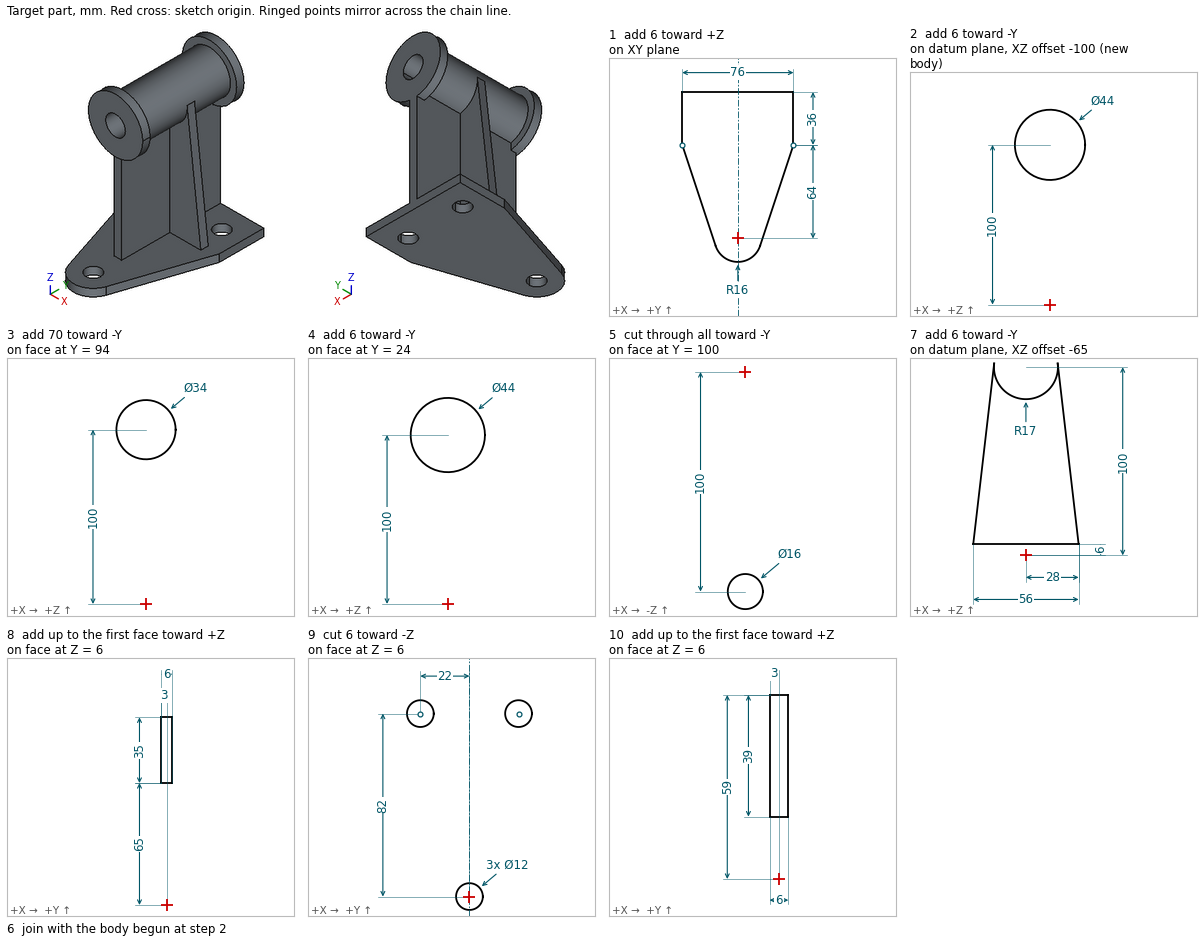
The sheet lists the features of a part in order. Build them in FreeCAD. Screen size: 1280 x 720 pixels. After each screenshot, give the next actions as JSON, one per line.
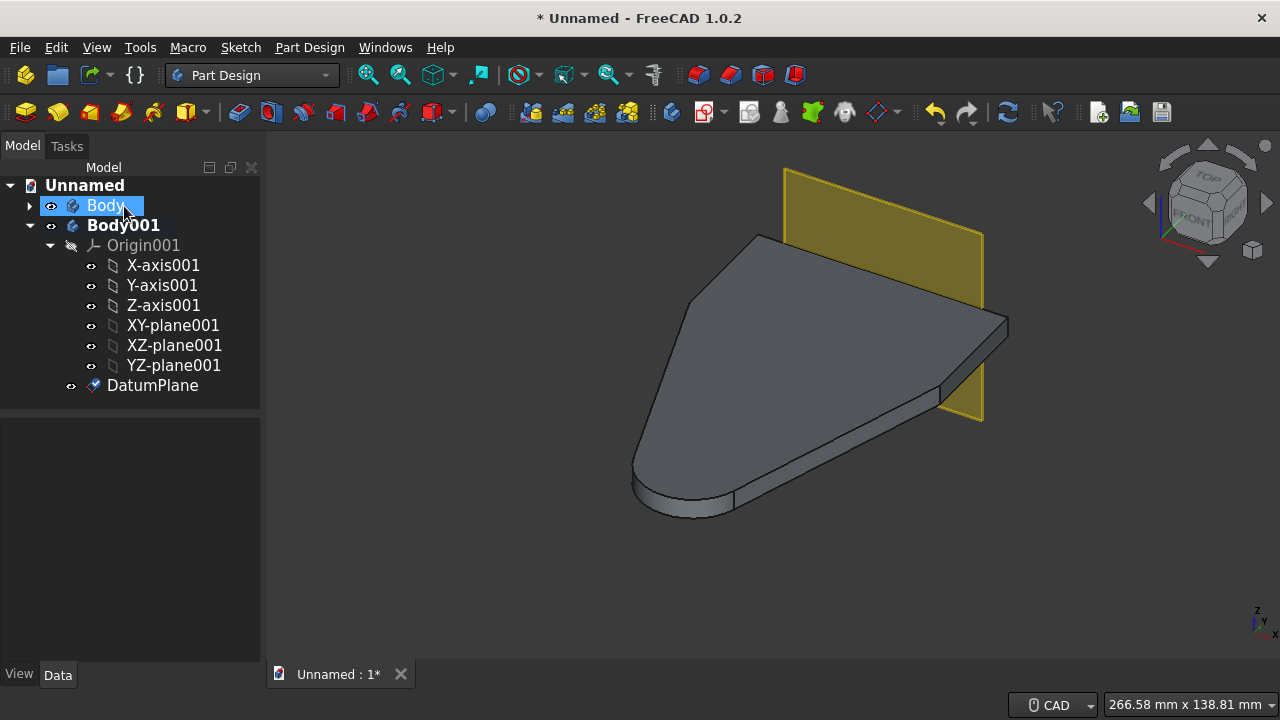
{"action": "left_click", "coordinate": [116, 386]}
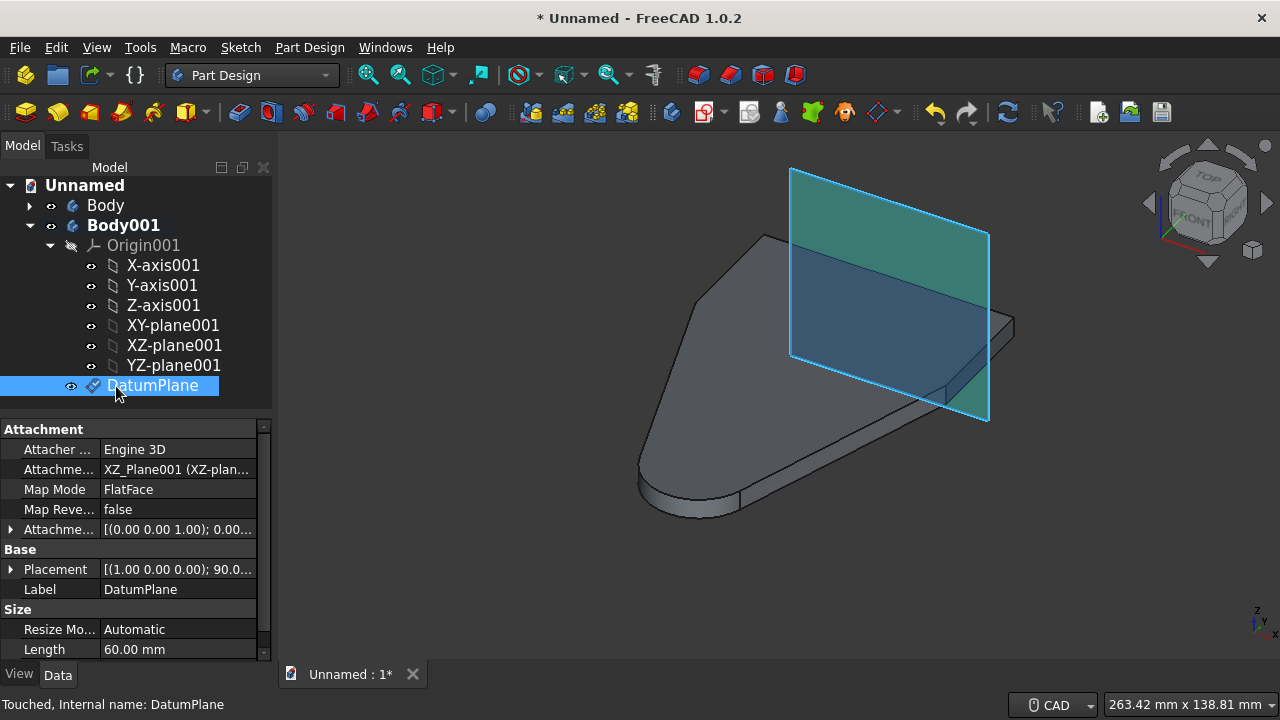
{"action": "left_click", "coordinate": [704, 112]}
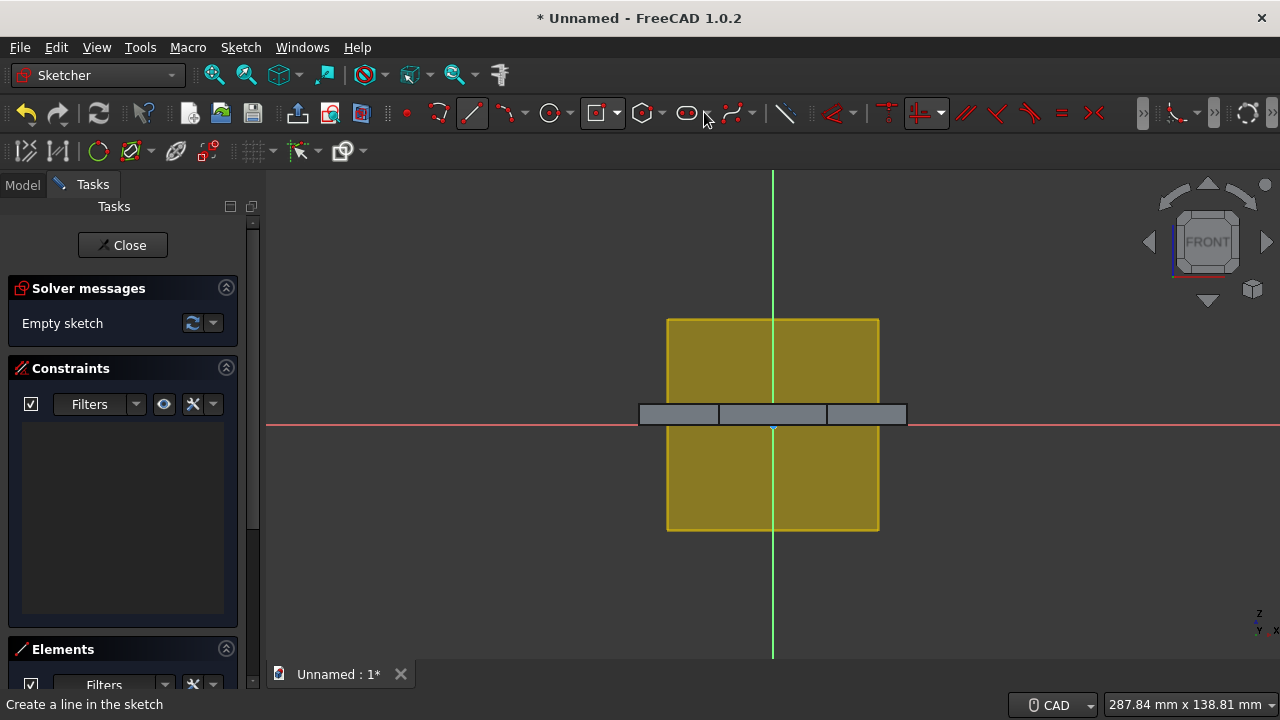
{"action": "scroll", "coordinate": [704, 414], "scroll_direction": "down", "scroll_amount": 5}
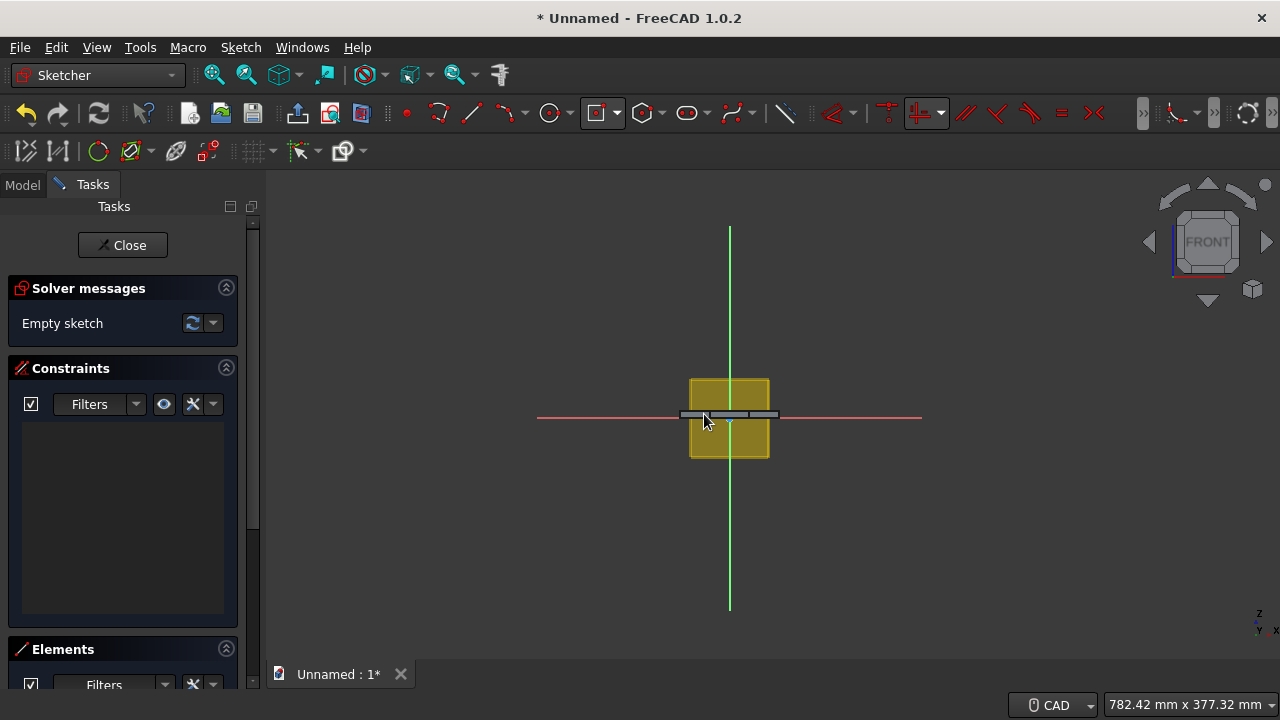
{"action": "scroll", "coordinate": [736, 257], "scroll_direction": "up", "scroll_amount": 8}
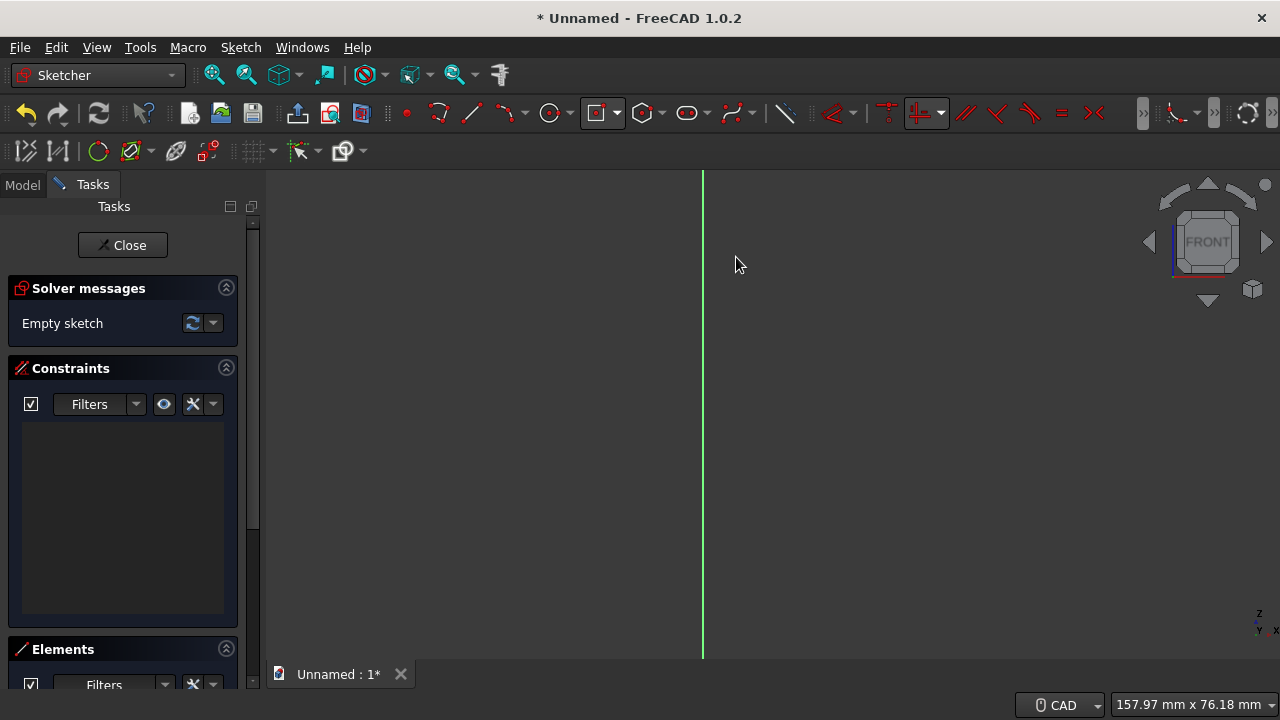
{"action": "key", "text": "g c"}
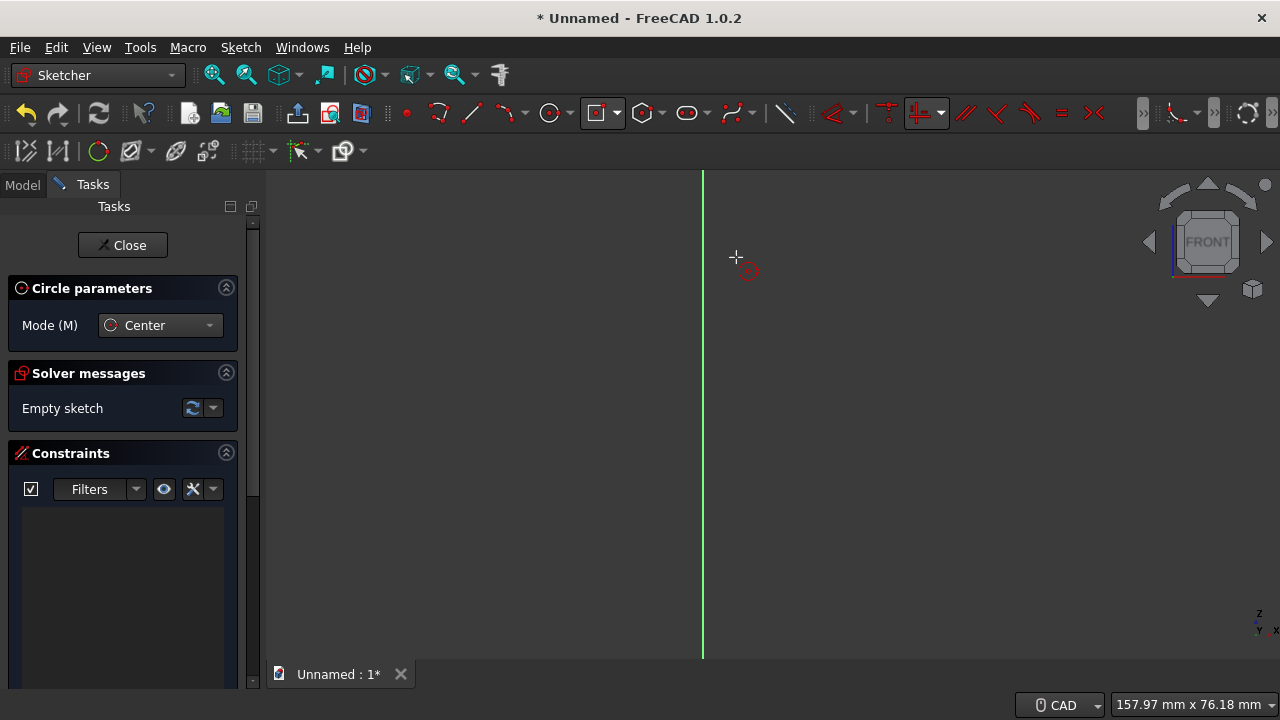
{"action": "left_click", "coordinate": [703, 414]}
{"action": "left_click", "coordinate": [803, 314]}
{"action": "key", "text": "Escape"}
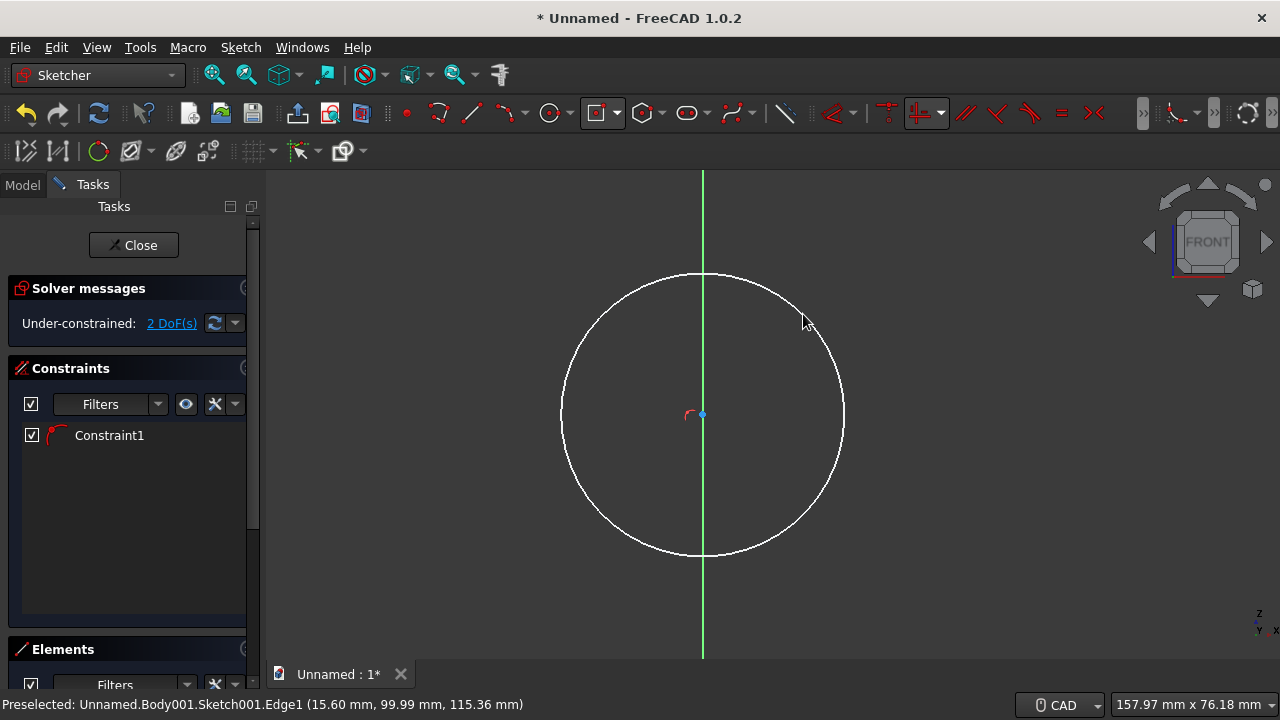
{"action": "key", "text": "d"}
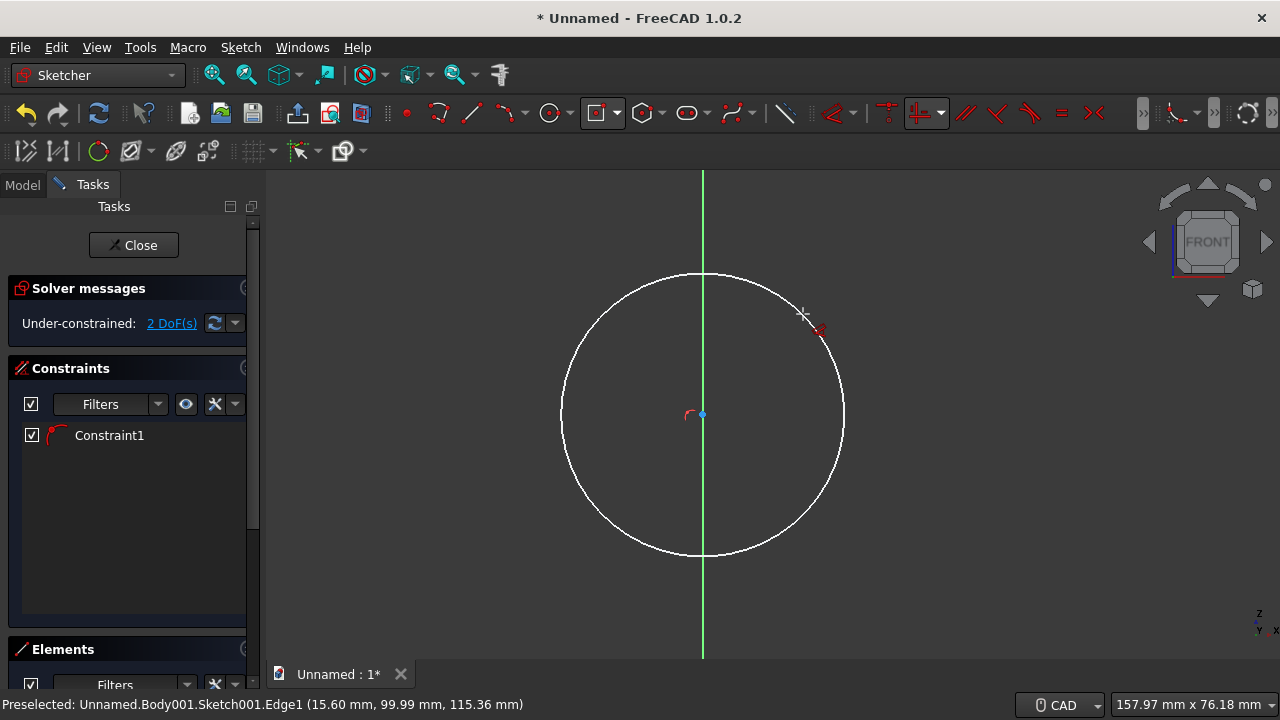
{"action": "left_click", "coordinate": [803, 315]}
{"action": "left_click", "coordinate": [826, 292]}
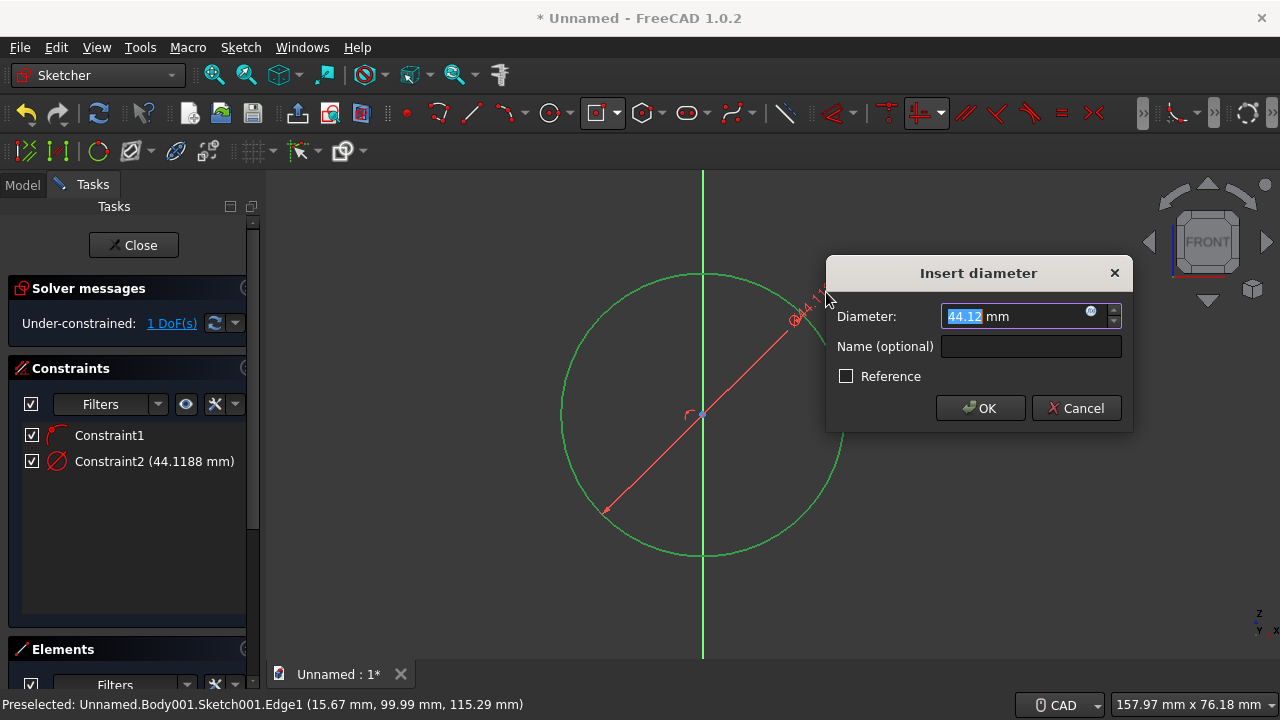
{"action": "type", "text": "44"}
{"action": "key", "text": "Return"}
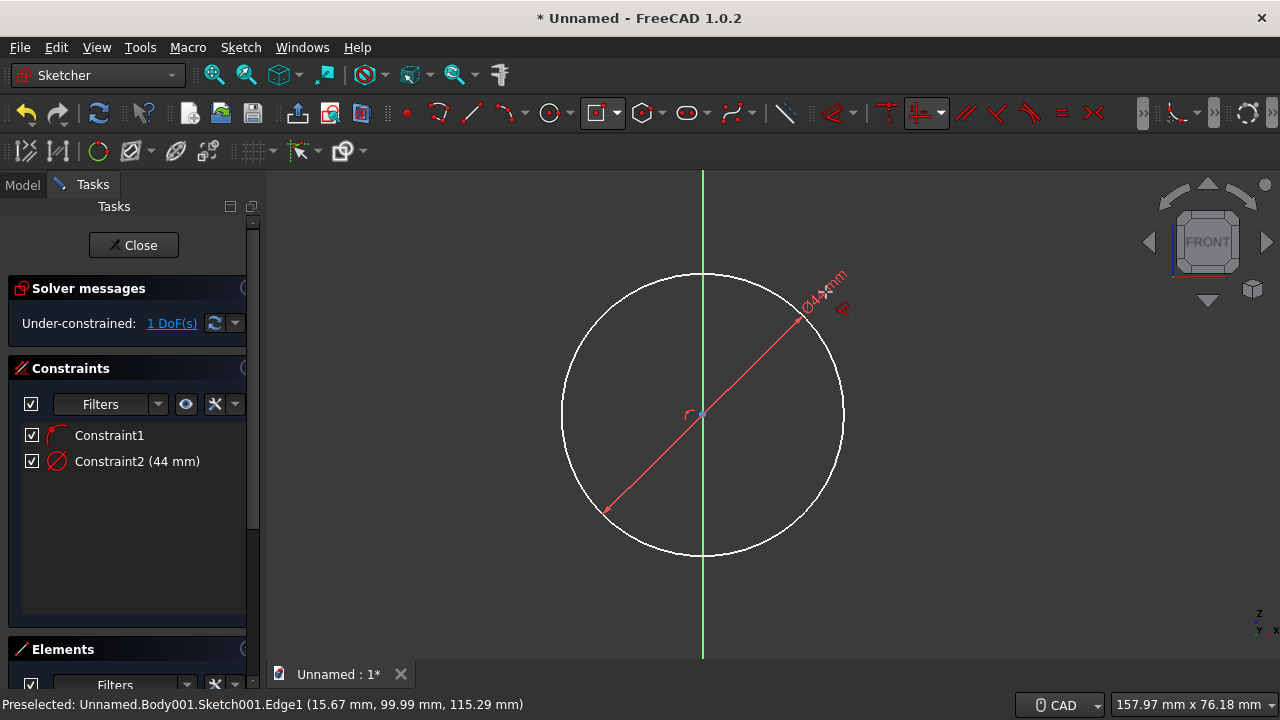
{"action": "left_click", "coordinate": [703, 415]}
{"action": "left_click", "coordinate": [737, 523]}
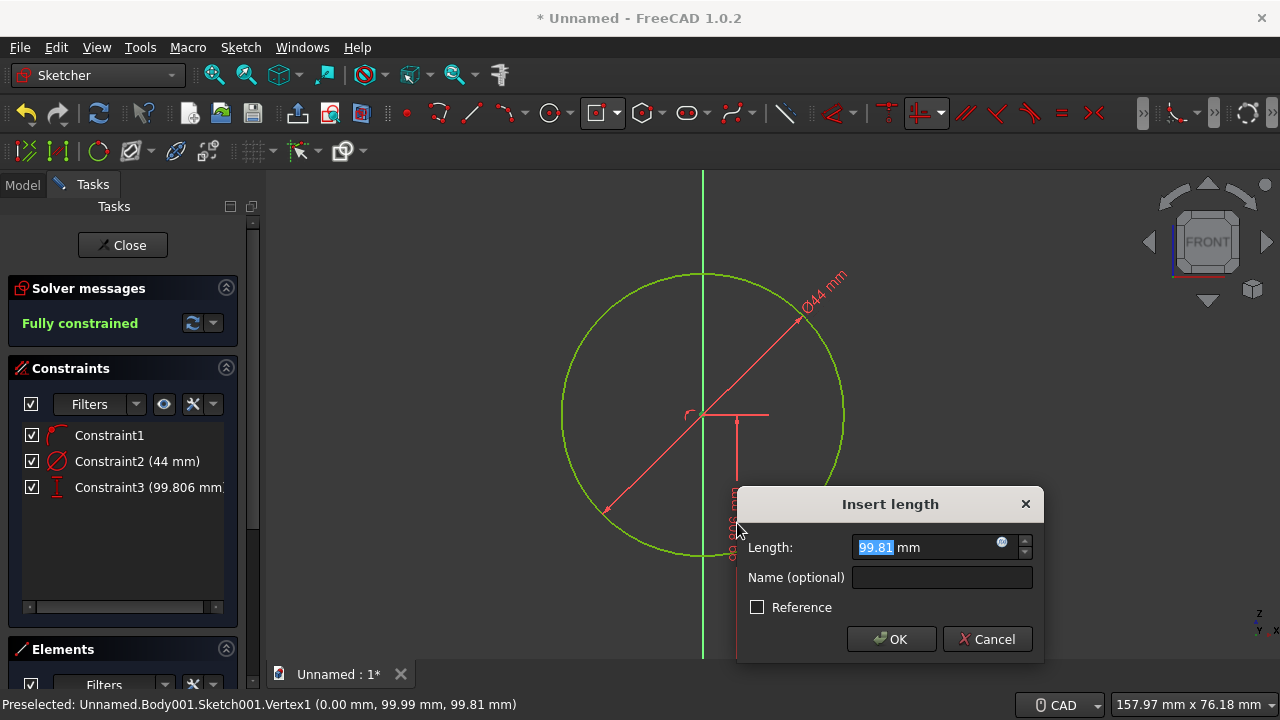
{"action": "type", "text": "100"}
{"action": "key", "text": "Return"}
{"action": "key", "text": "Escape"}